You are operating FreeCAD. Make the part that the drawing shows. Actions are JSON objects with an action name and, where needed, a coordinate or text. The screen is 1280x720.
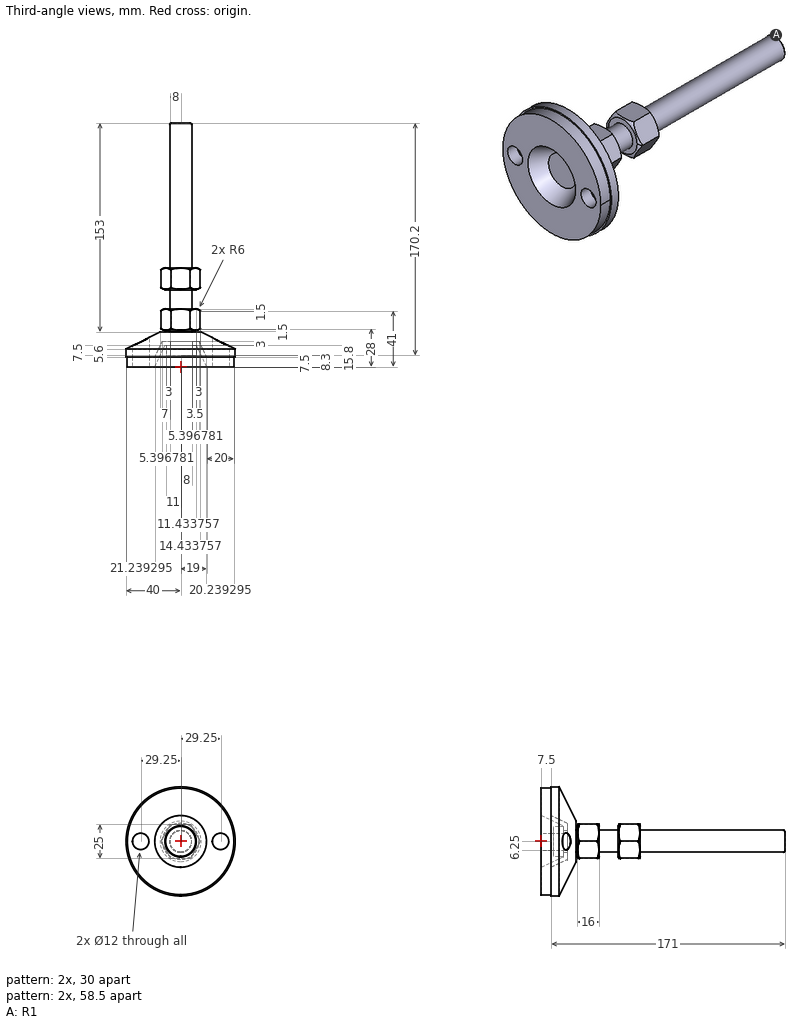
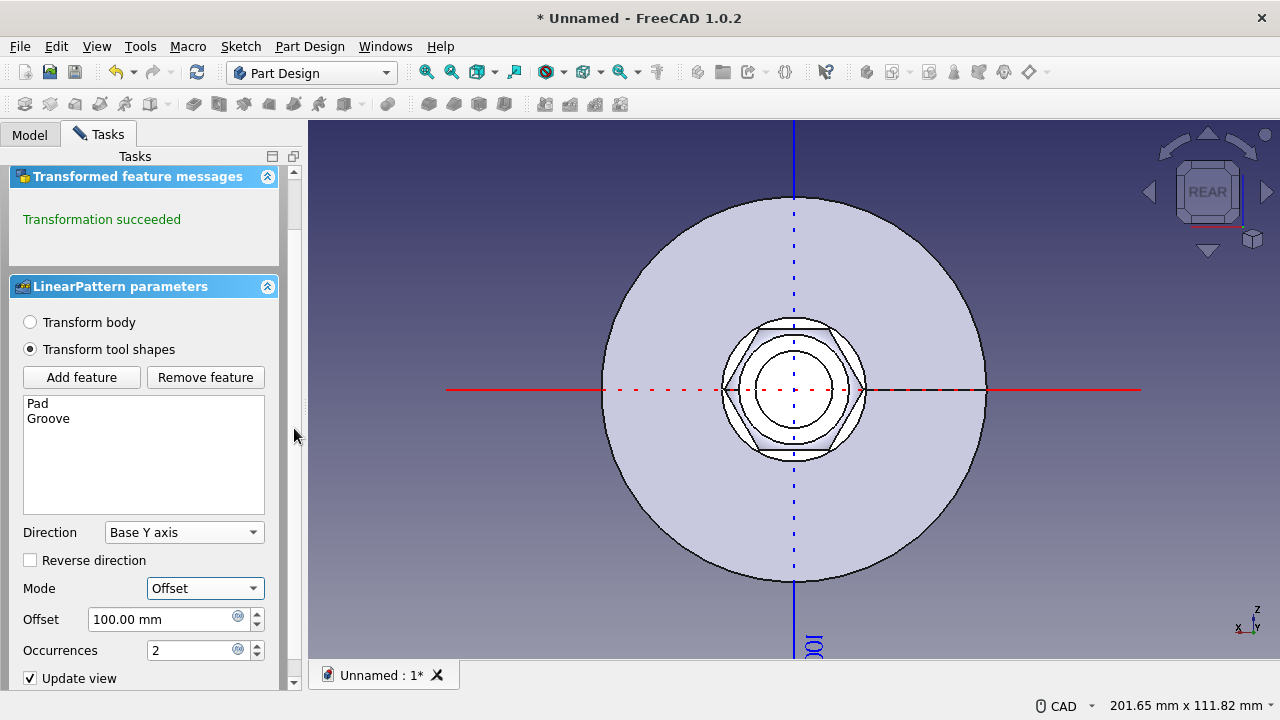
{"action": "triple_click", "coordinate": [170, 598]}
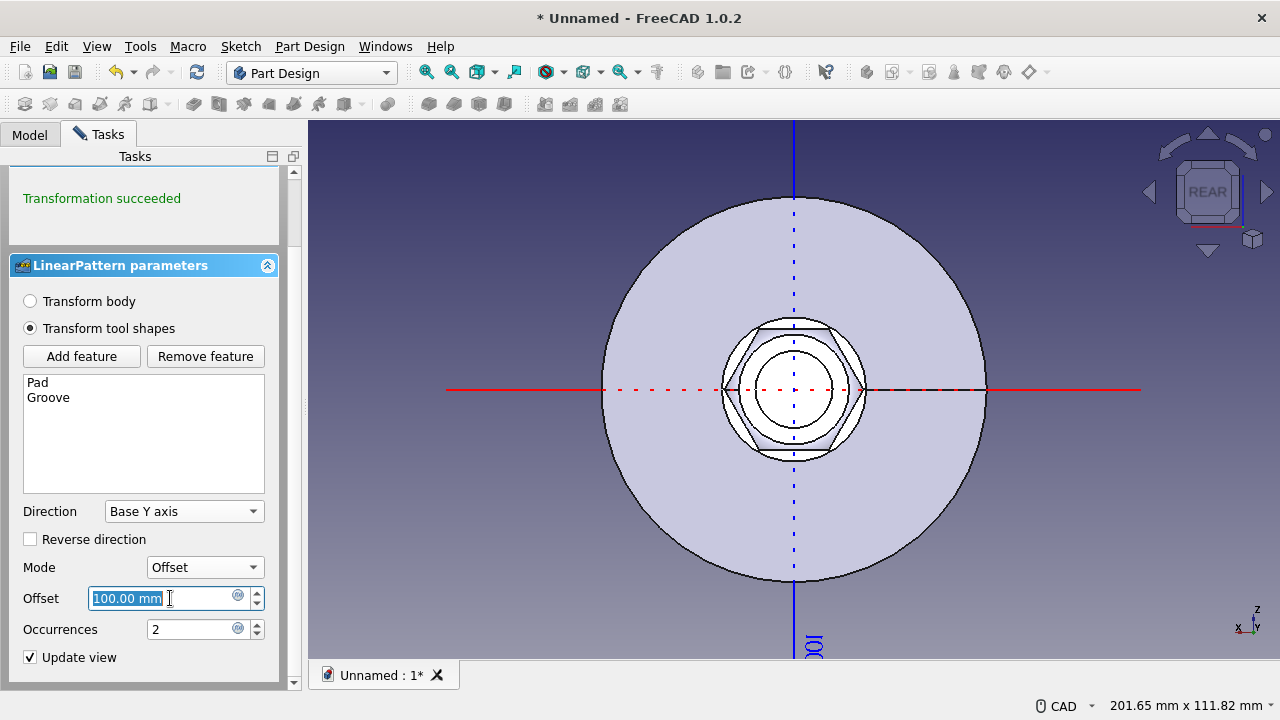
{"action": "type", "text": "30"}
{"action": "key", "text": "Tab"}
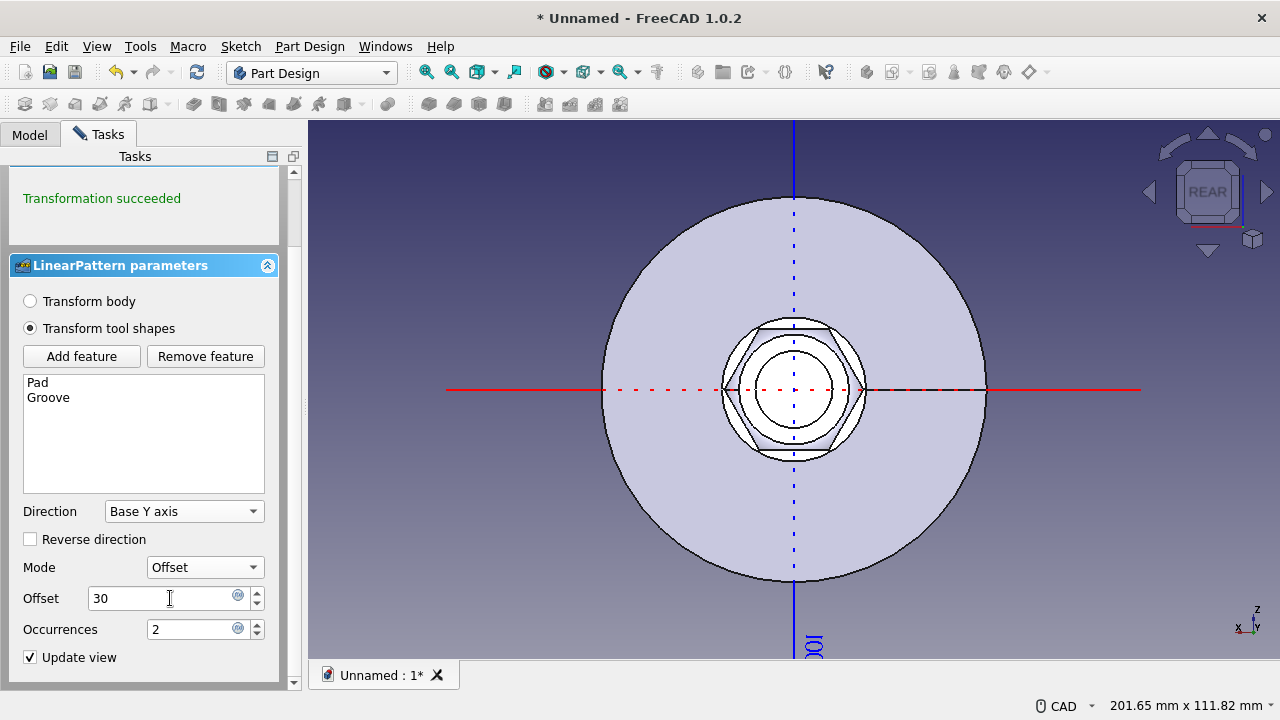
{"action": "triple_click", "coordinate": [199, 630]}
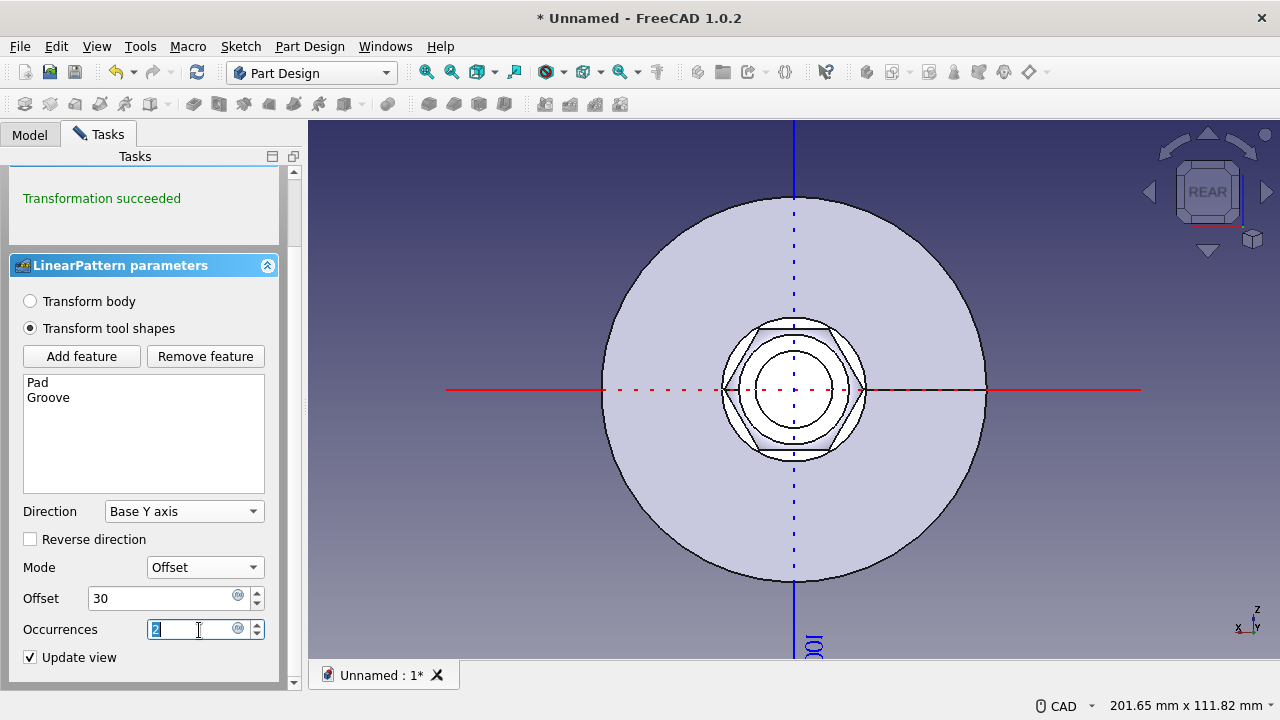
{"action": "type", "text": "2"}
{"action": "key", "text": "Tab"}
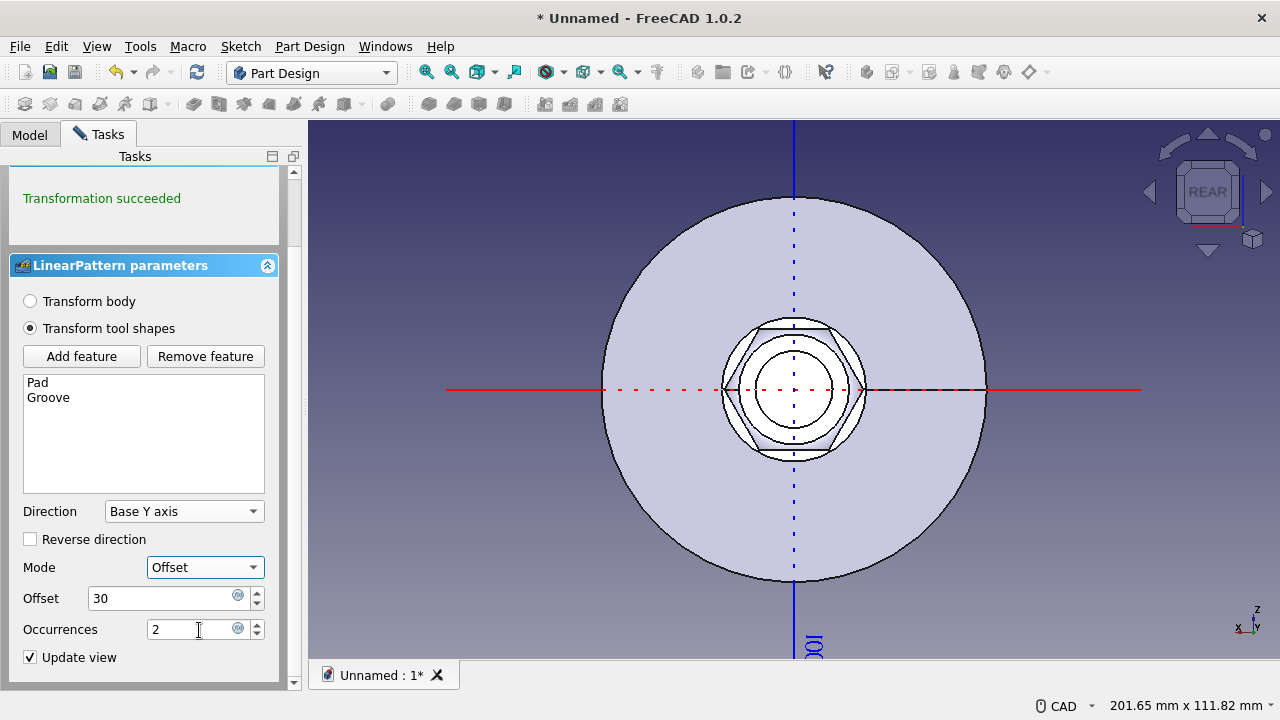
{"action": "scroll", "coordinate": [294, 428], "scroll_direction": "up", "scroll_amount": 3}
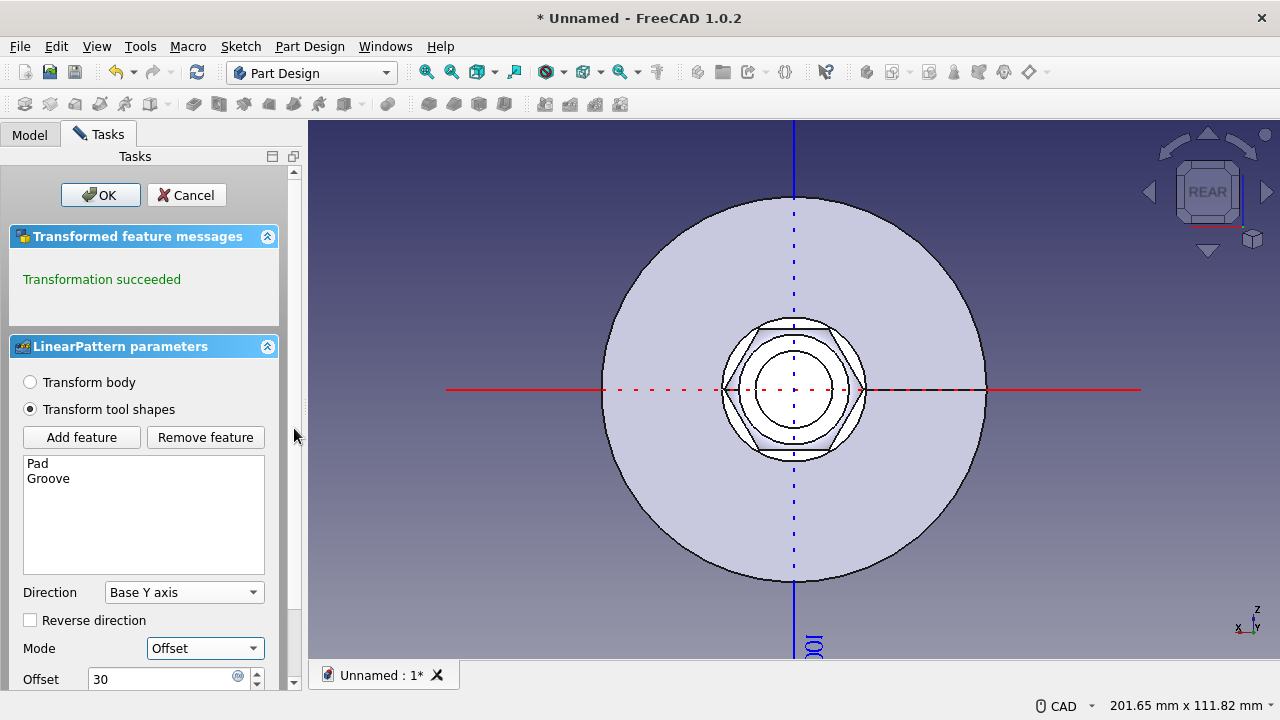
{"action": "left_click", "coordinate": [101, 195]}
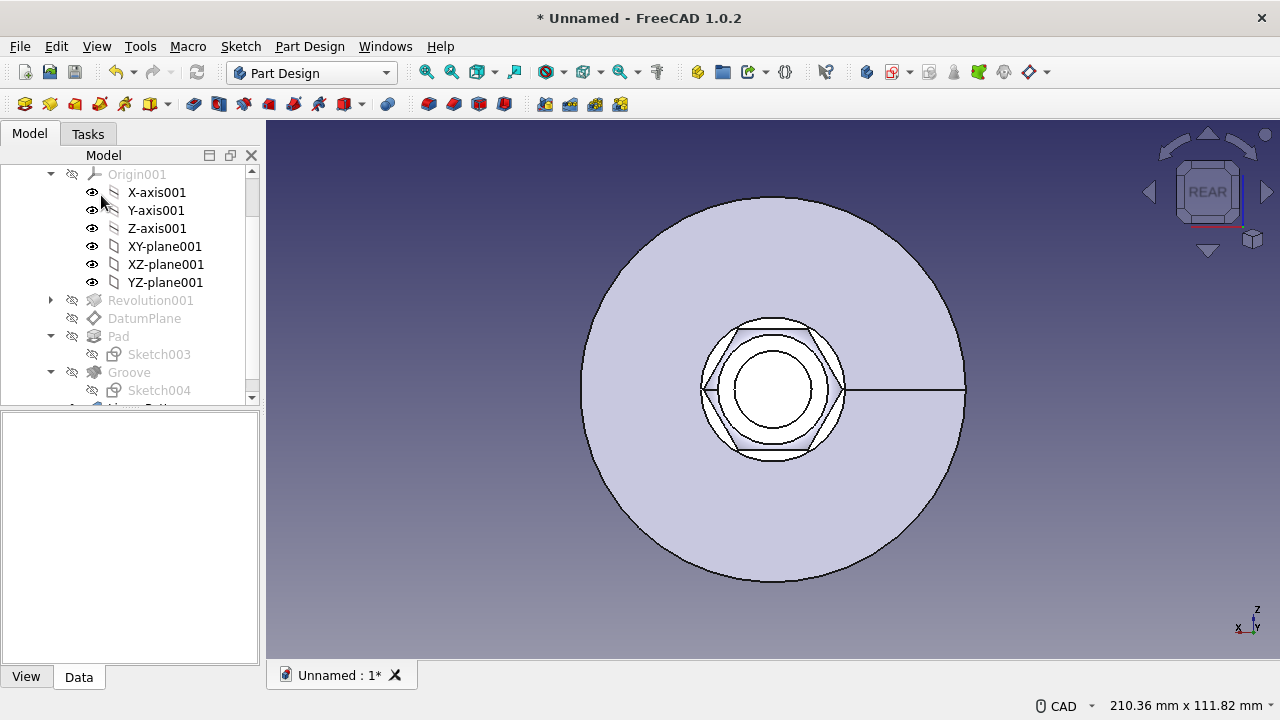
{"action": "left_click", "coordinate": [137, 282]}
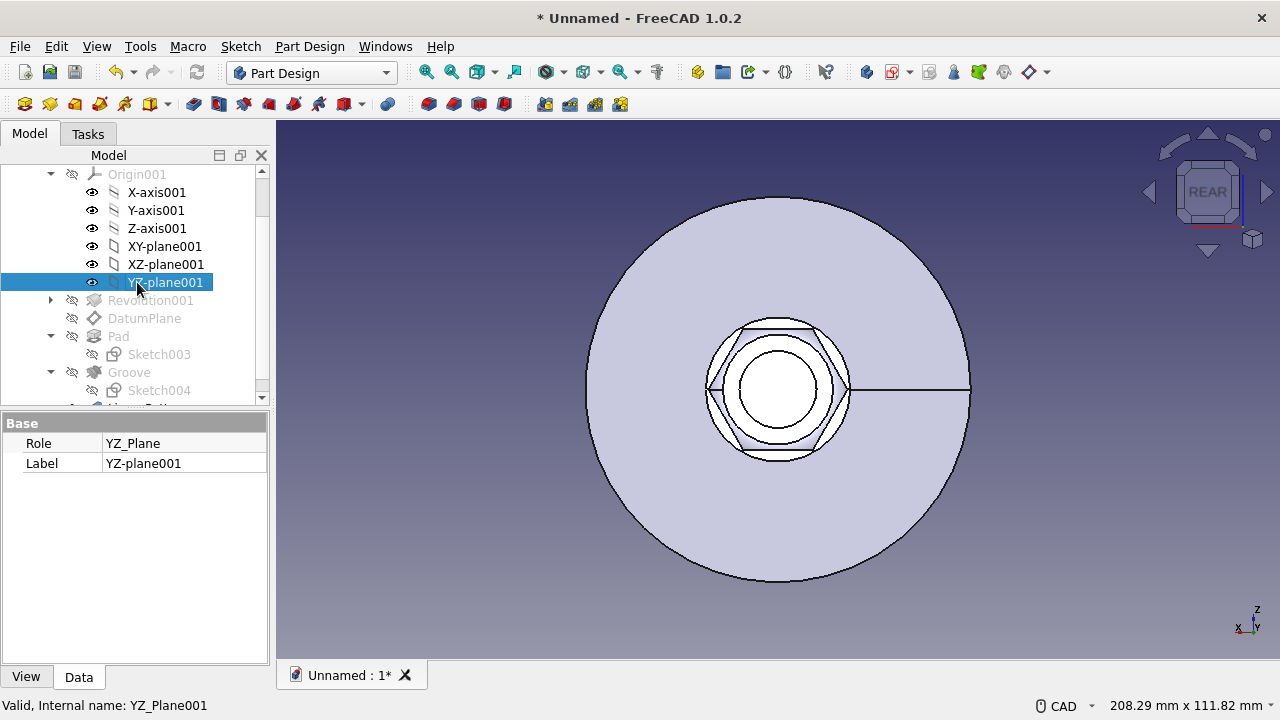
{"action": "left_click", "coordinate": [1028, 72]}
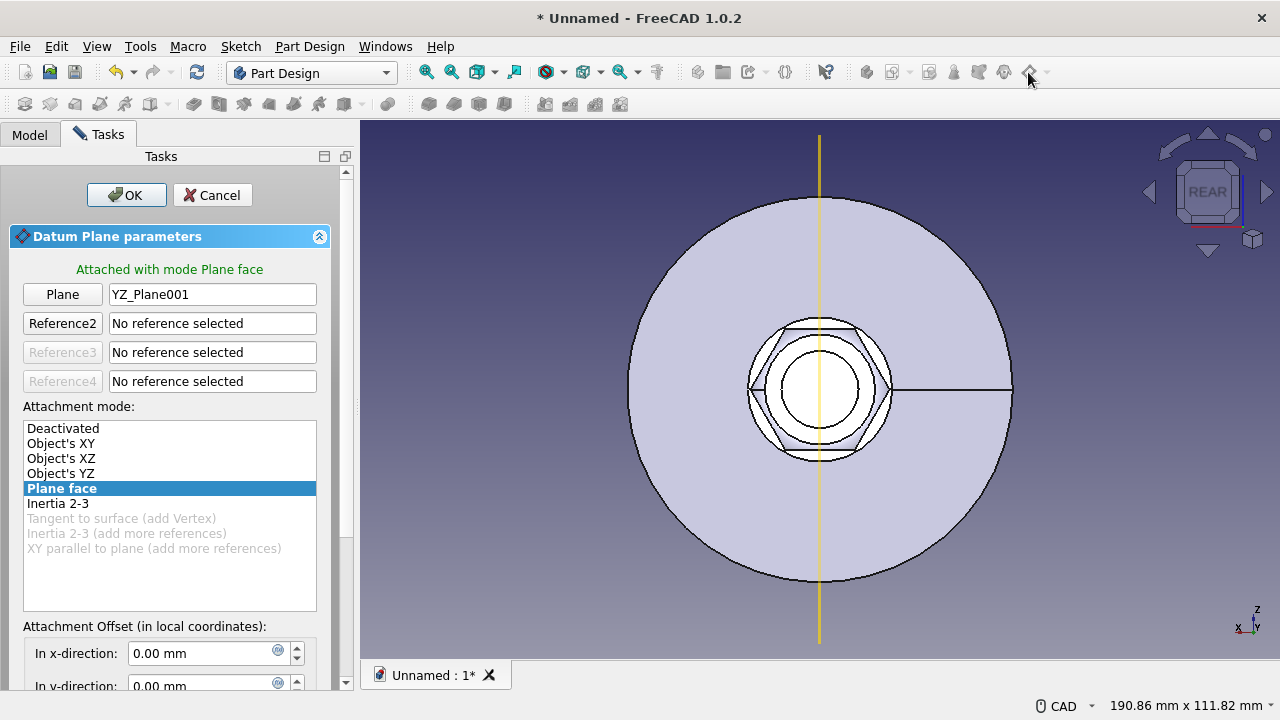
{"action": "scroll", "coordinate": [346, 428], "scroll_direction": "down", "scroll_amount": 2}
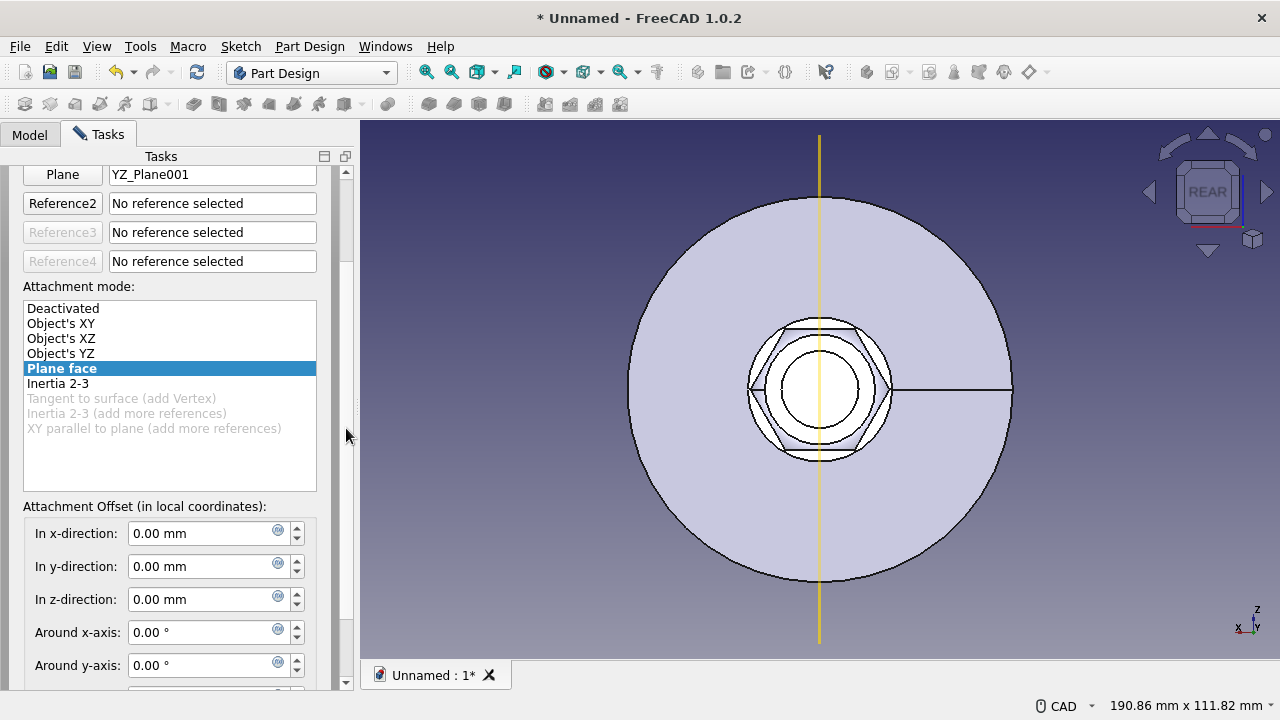
{"action": "triple_click", "coordinate": [210, 600]}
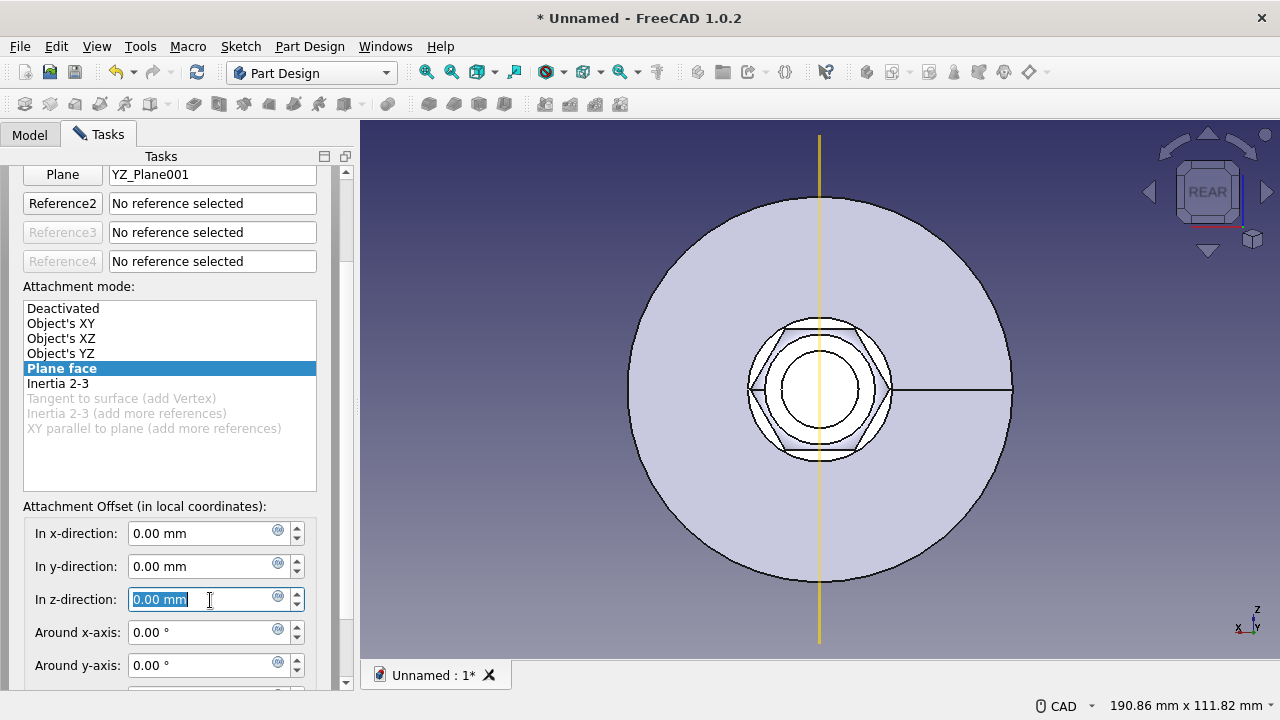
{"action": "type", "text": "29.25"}
{"action": "key", "text": "Tab"}